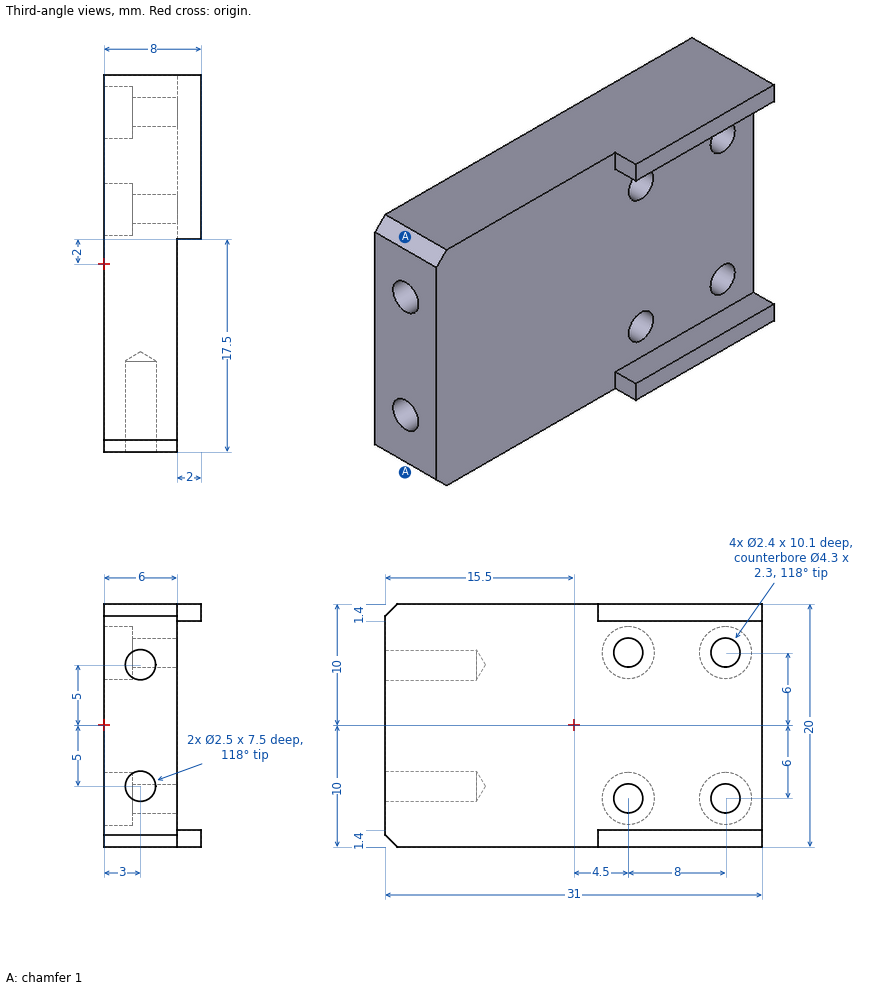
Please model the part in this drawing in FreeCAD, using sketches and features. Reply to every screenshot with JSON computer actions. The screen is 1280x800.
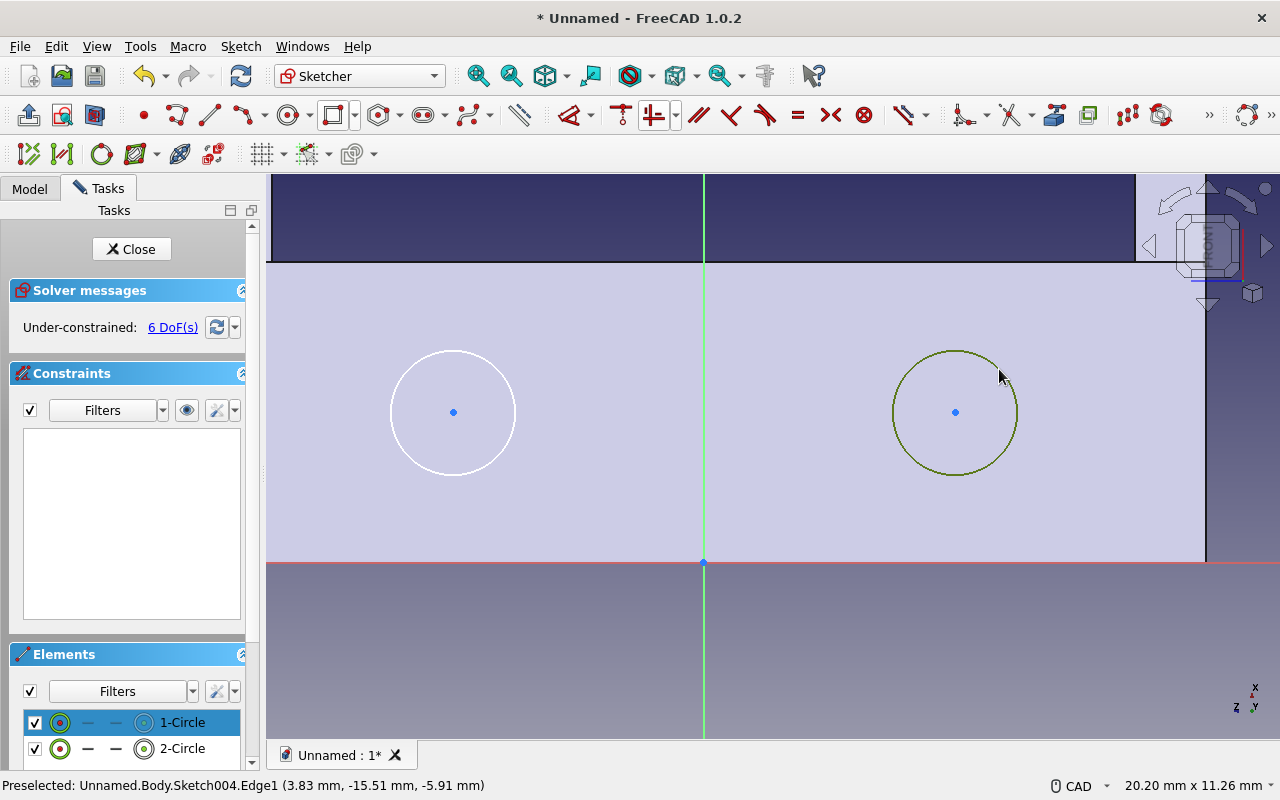
{"action": "left_click", "coordinate": [497, 369]}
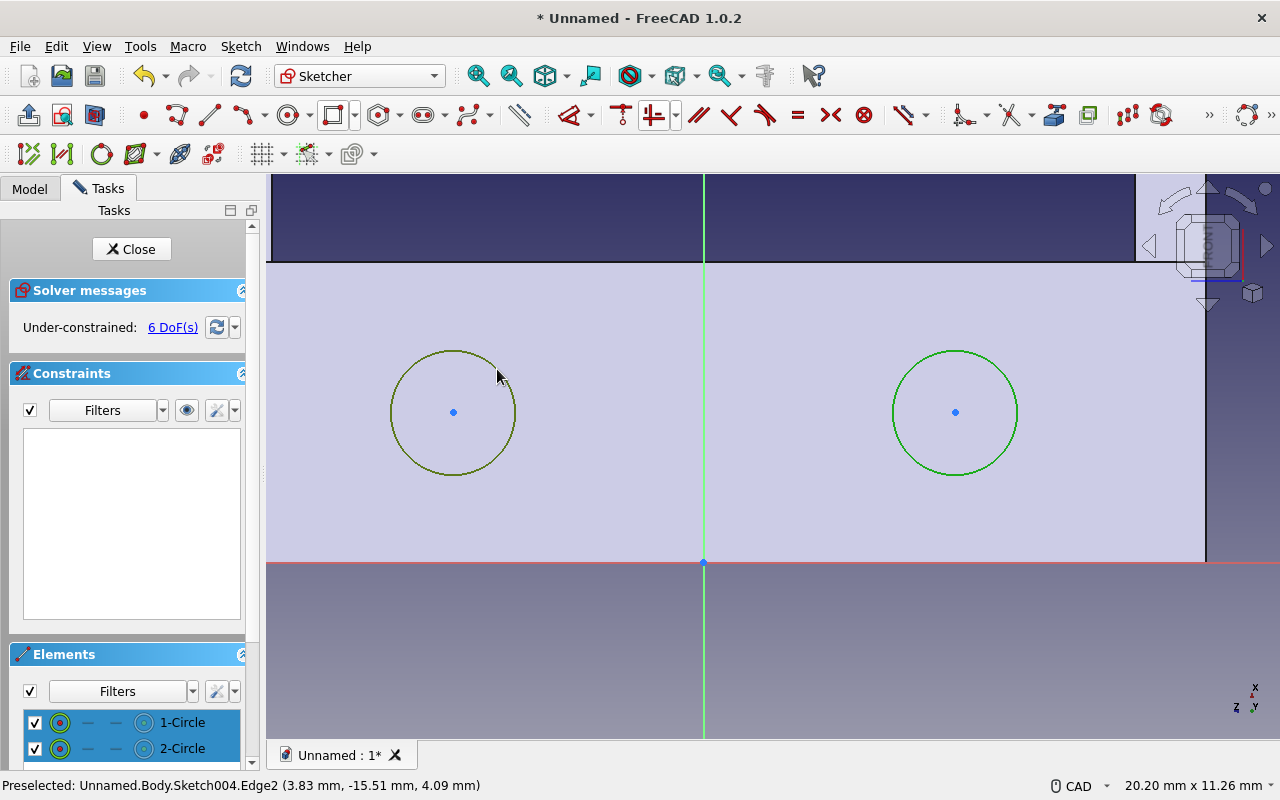
{"action": "left_click", "coordinate": [798, 116]}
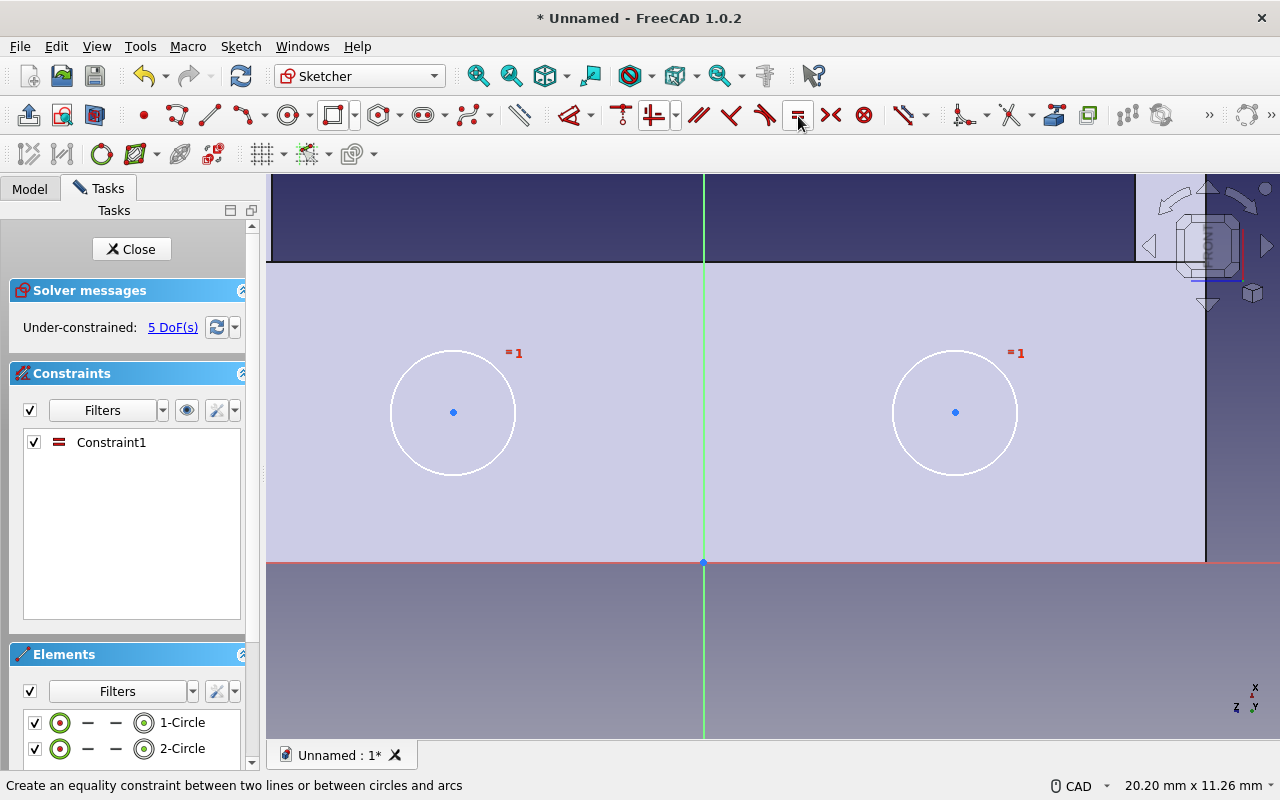
{"action": "left_click", "coordinate": [955, 413]}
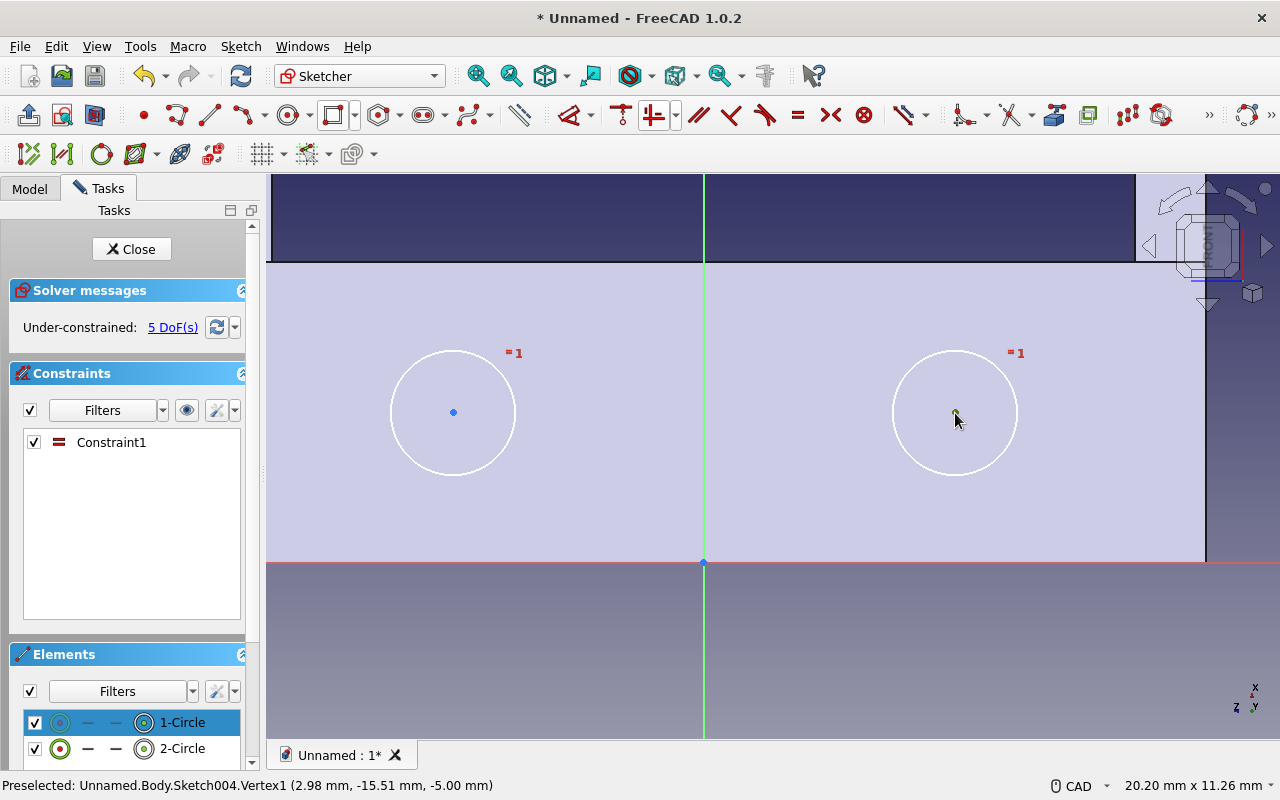
{"action": "left_click", "coordinate": [453, 413]}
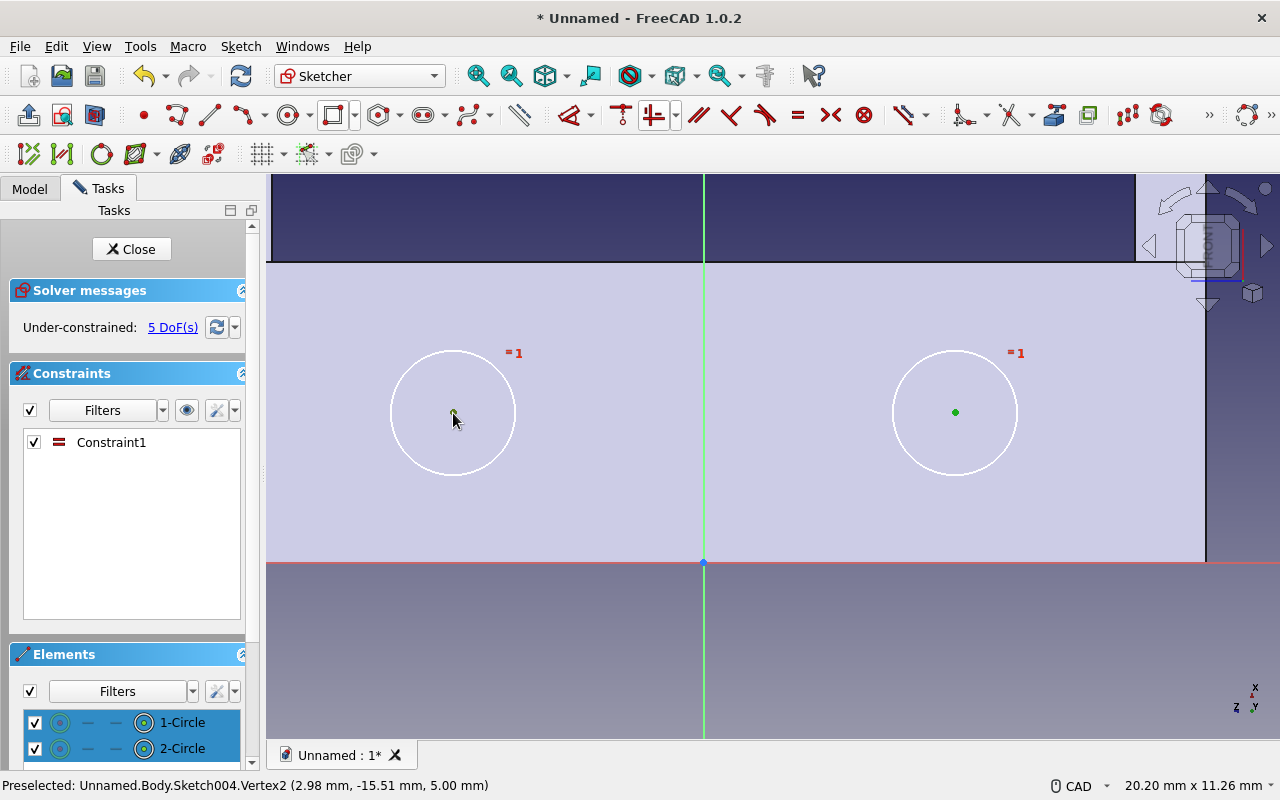
{"action": "left_click", "coordinate": [676, 116]}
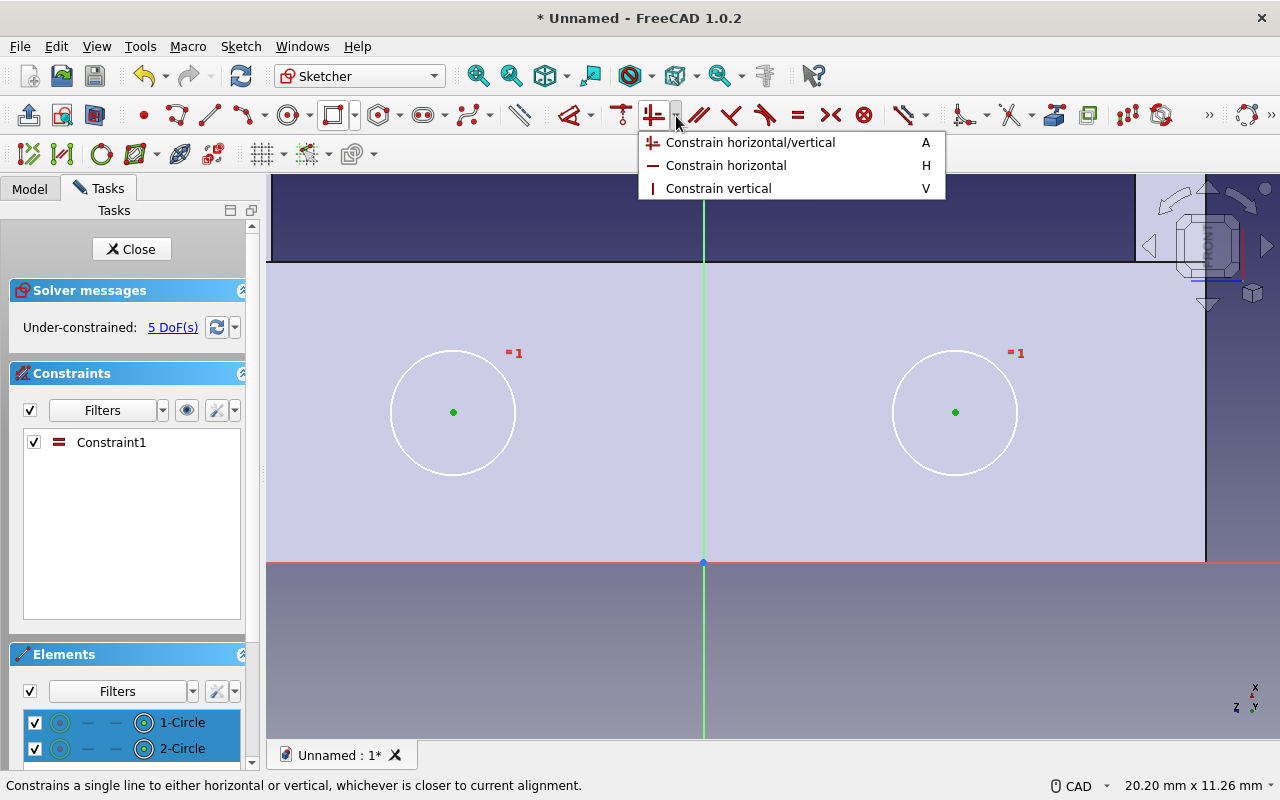
{"action": "left_click", "coordinate": [792, 166]}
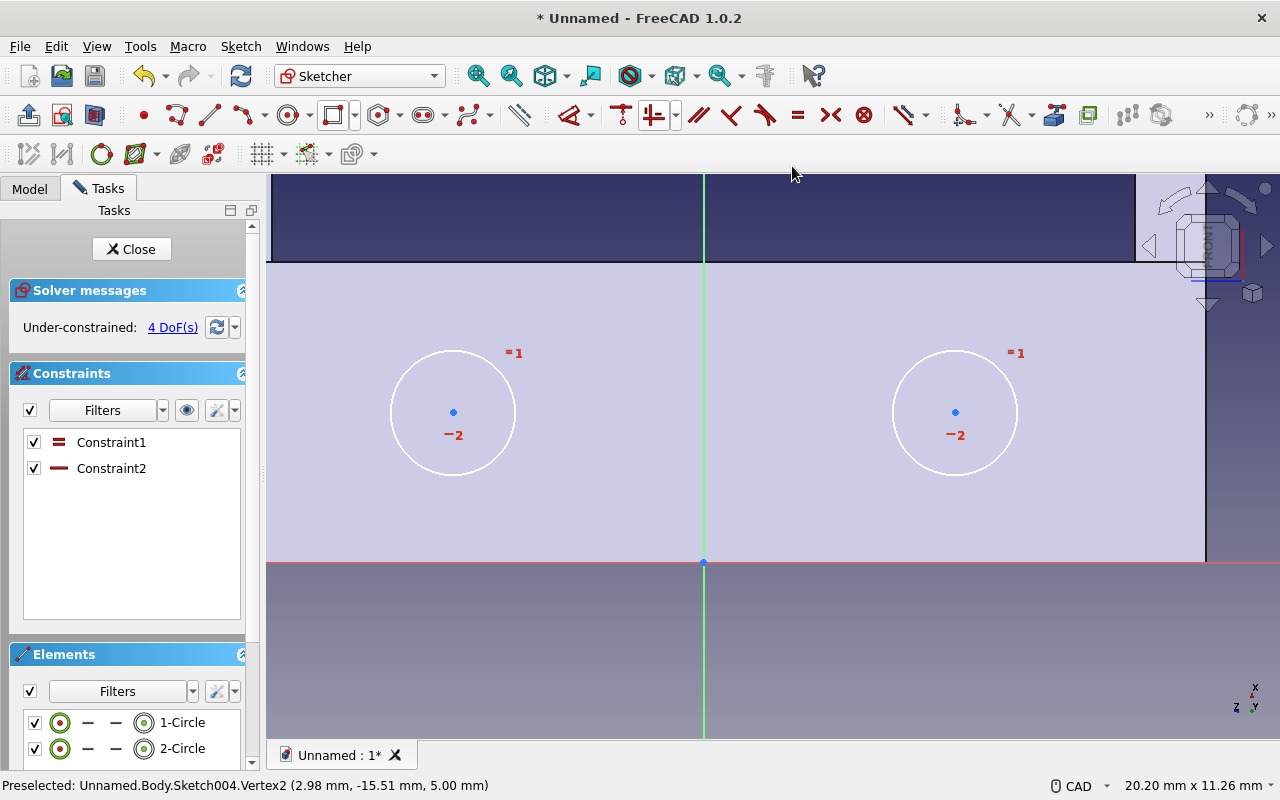
{"action": "left_click", "coordinate": [568, 116]}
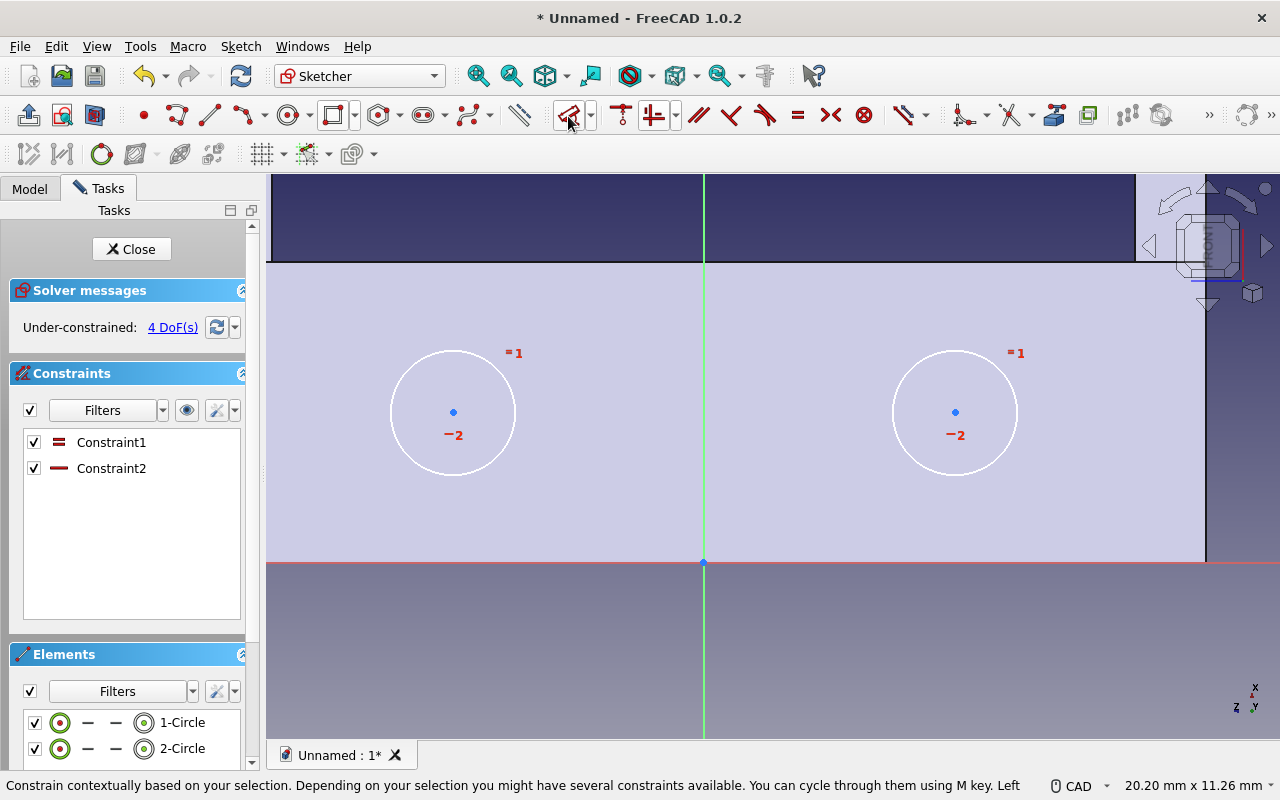
{"action": "left_click", "coordinate": [999, 369]}
{"action": "left_click", "coordinate": [1022, 346]}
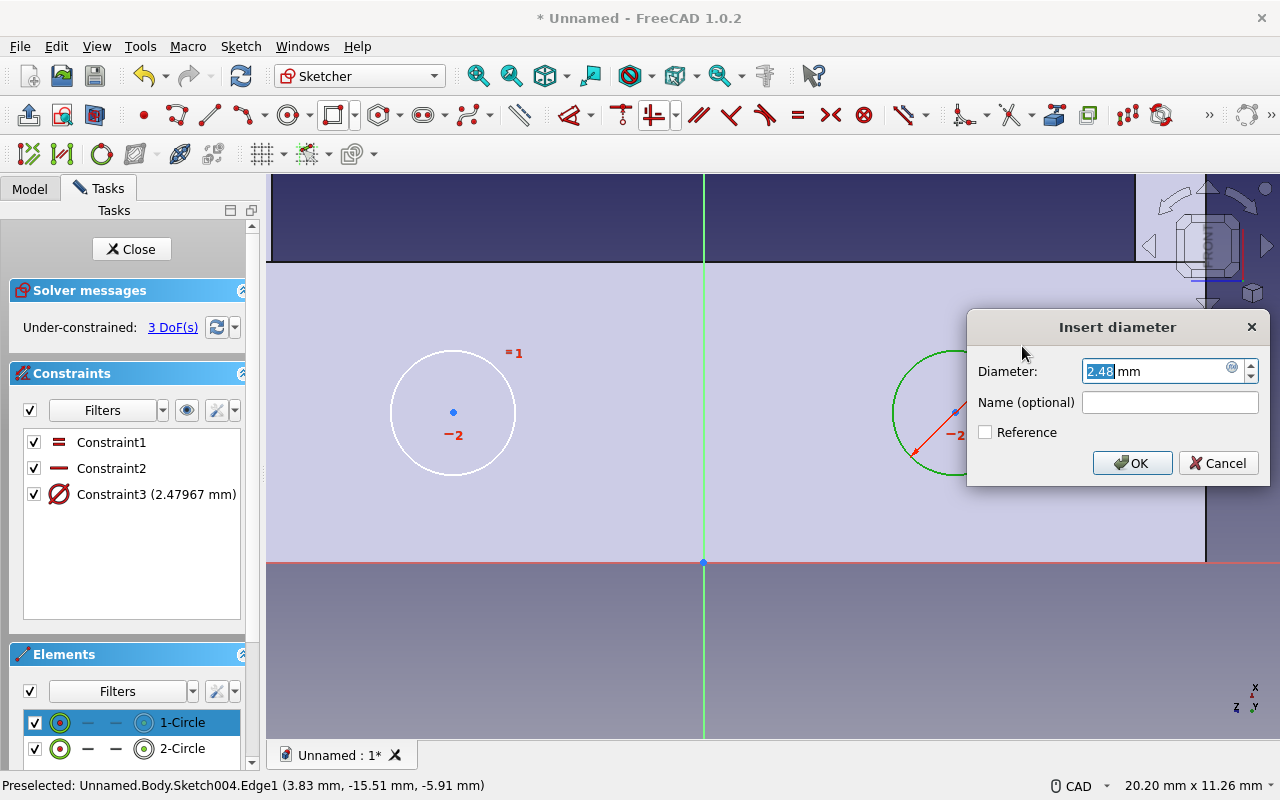
{"action": "type", "text": "2.5"}
{"action": "key", "text": "Return"}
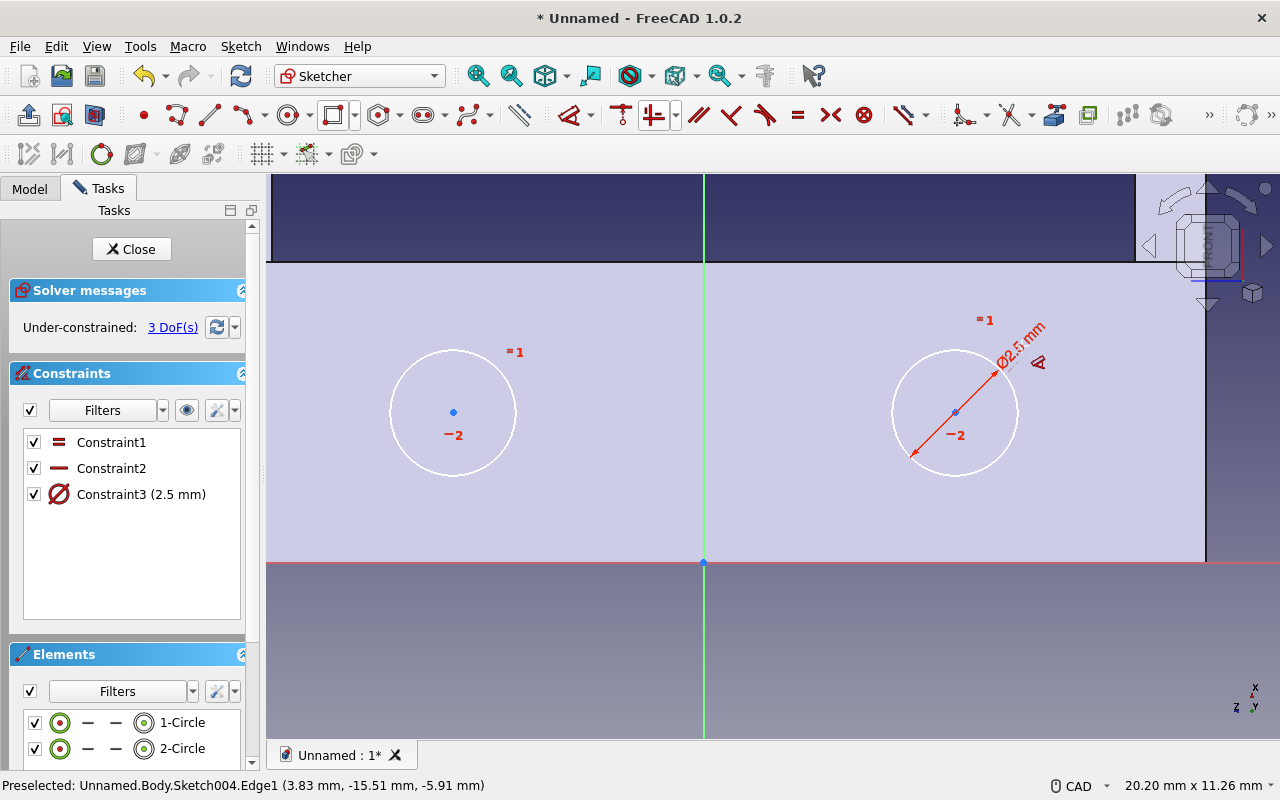
{"action": "left_click", "coordinate": [955, 413]}
{"action": "left_click", "coordinate": [829, 597]}